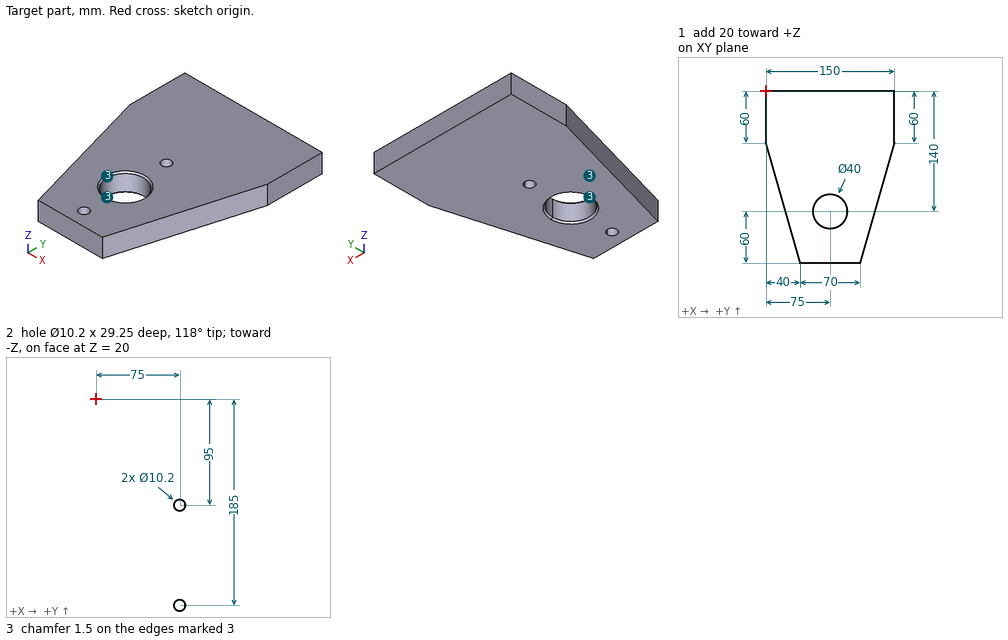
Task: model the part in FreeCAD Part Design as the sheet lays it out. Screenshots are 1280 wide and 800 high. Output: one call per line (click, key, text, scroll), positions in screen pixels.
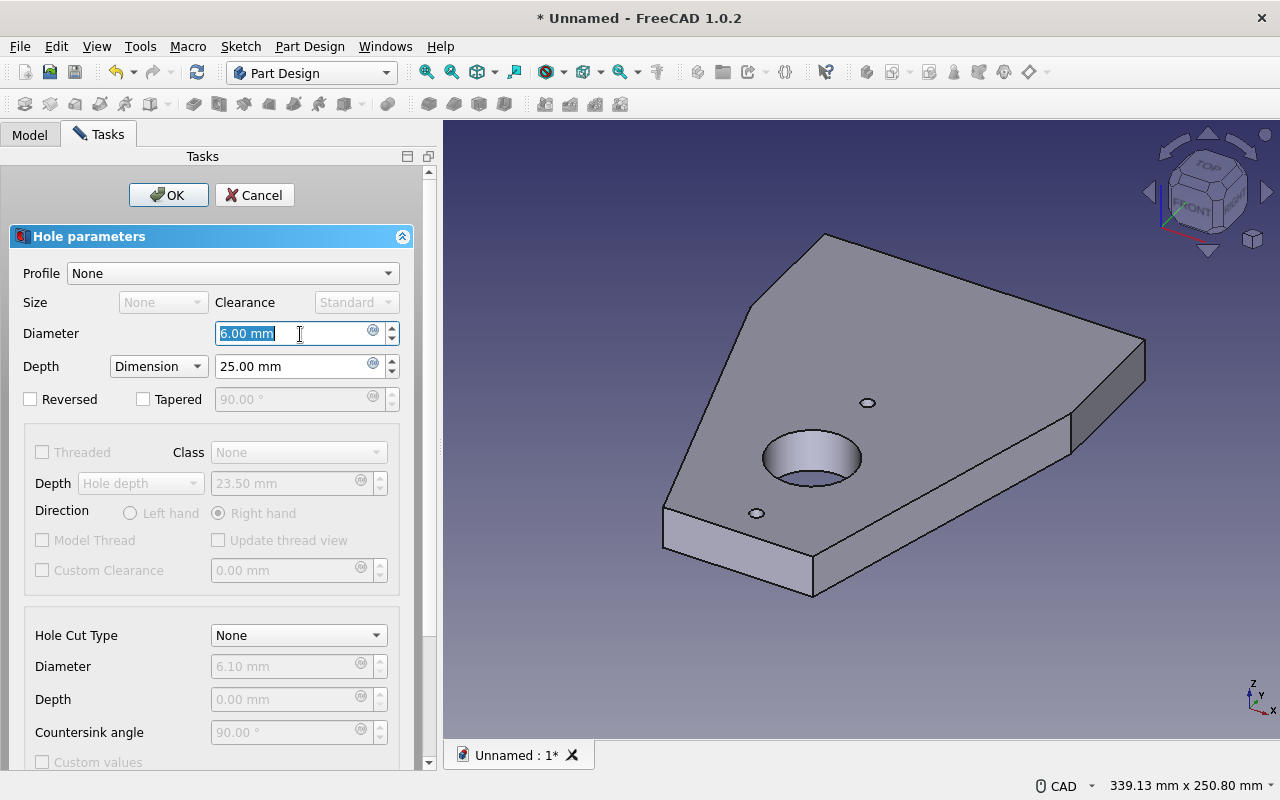
text(10.2)
key(Tab)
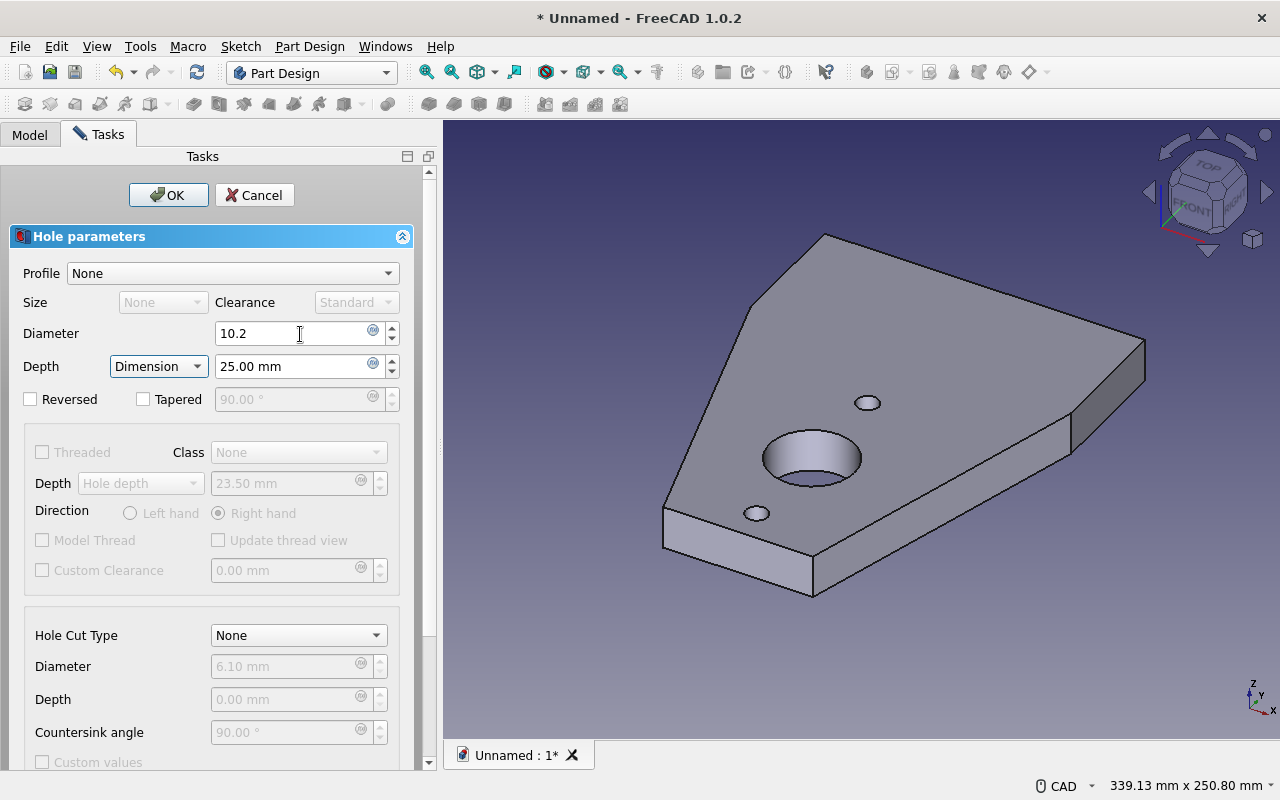
triple_click(300, 366)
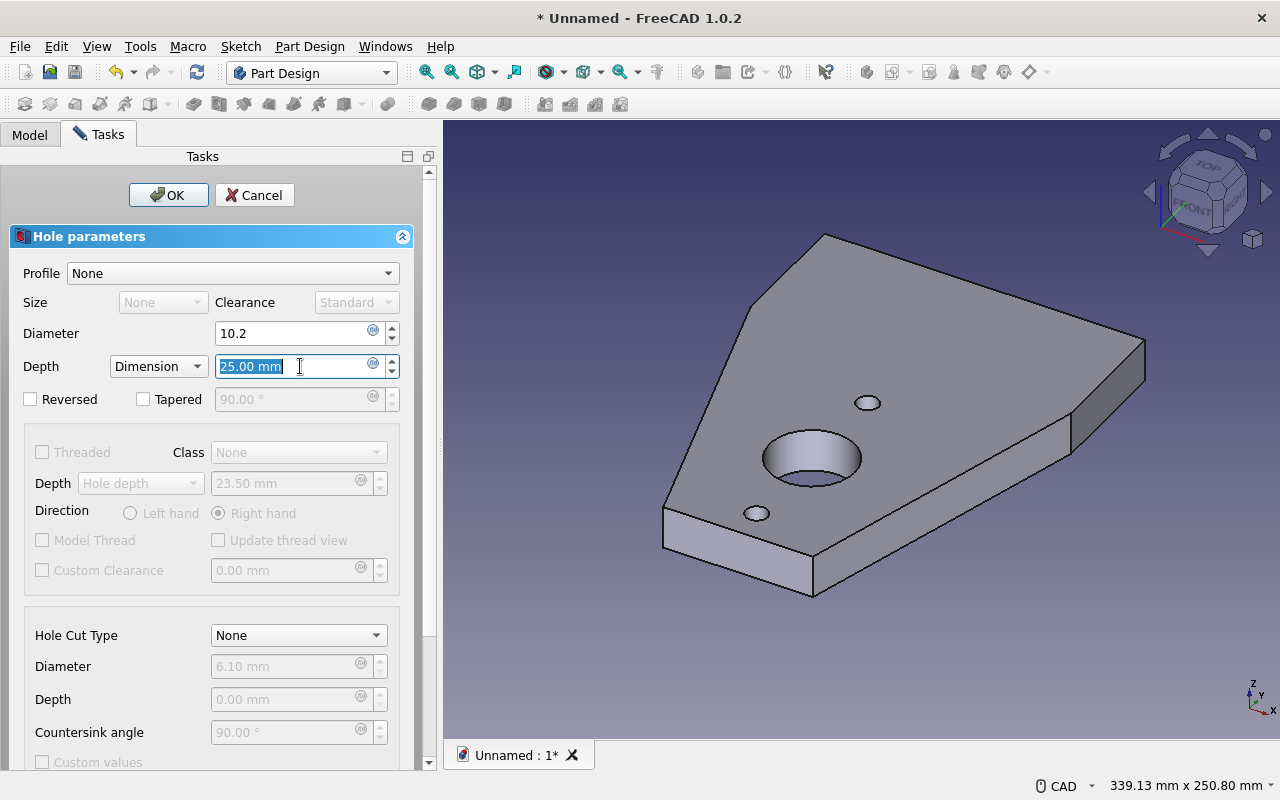
text(29.25)
key(Tab)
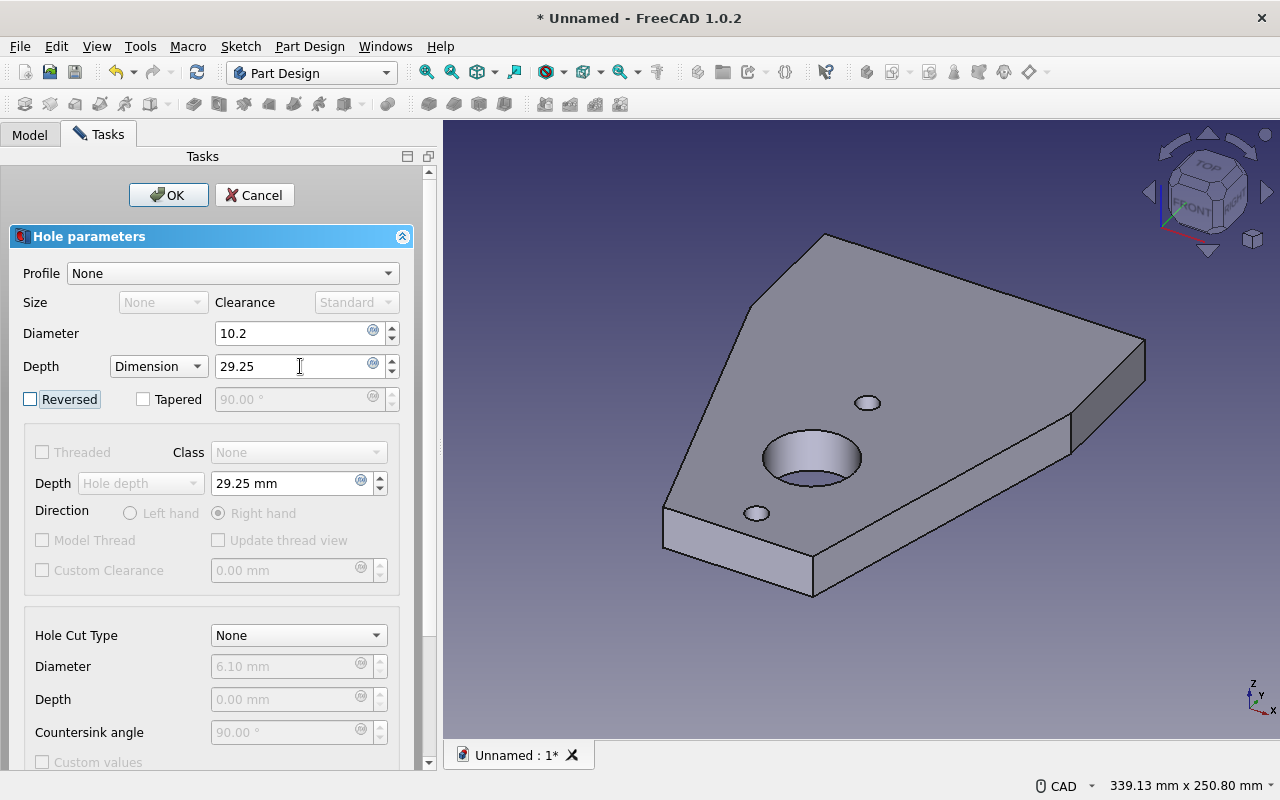
click(169, 195)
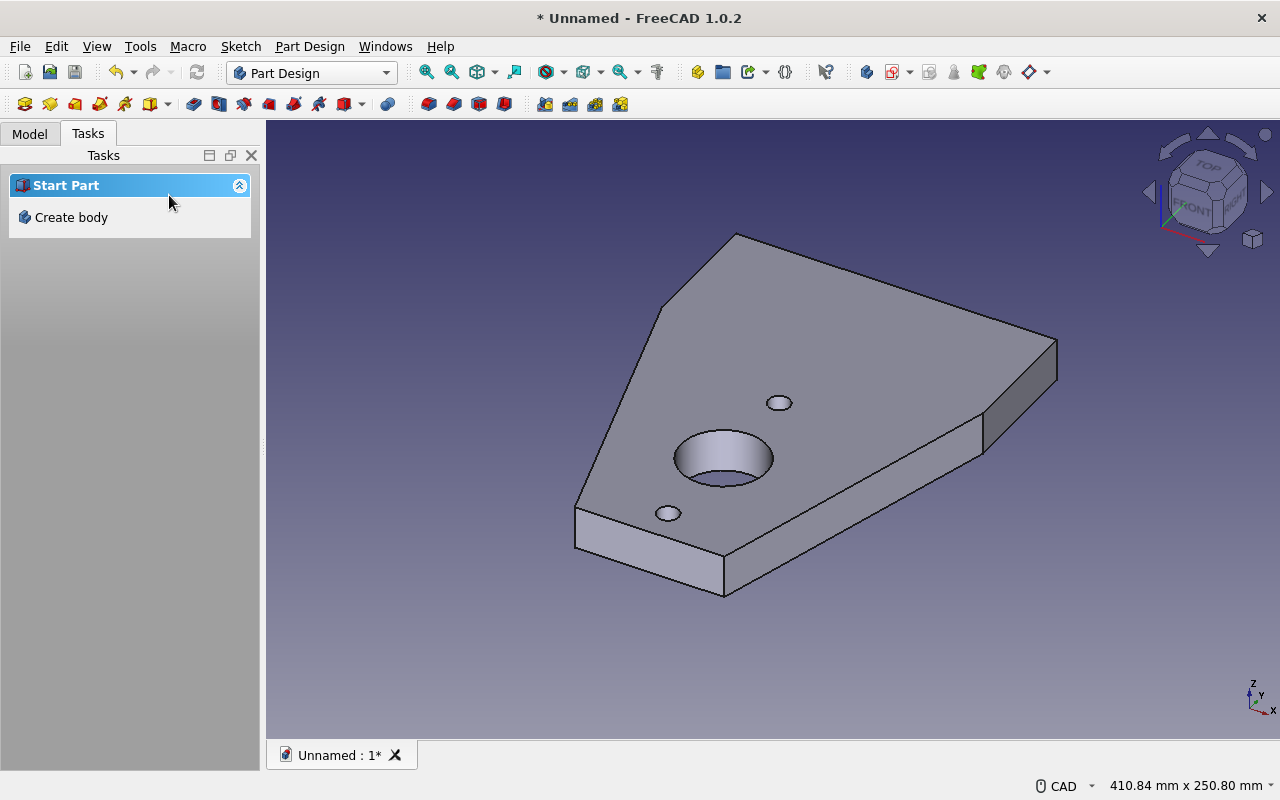
click(681, 443)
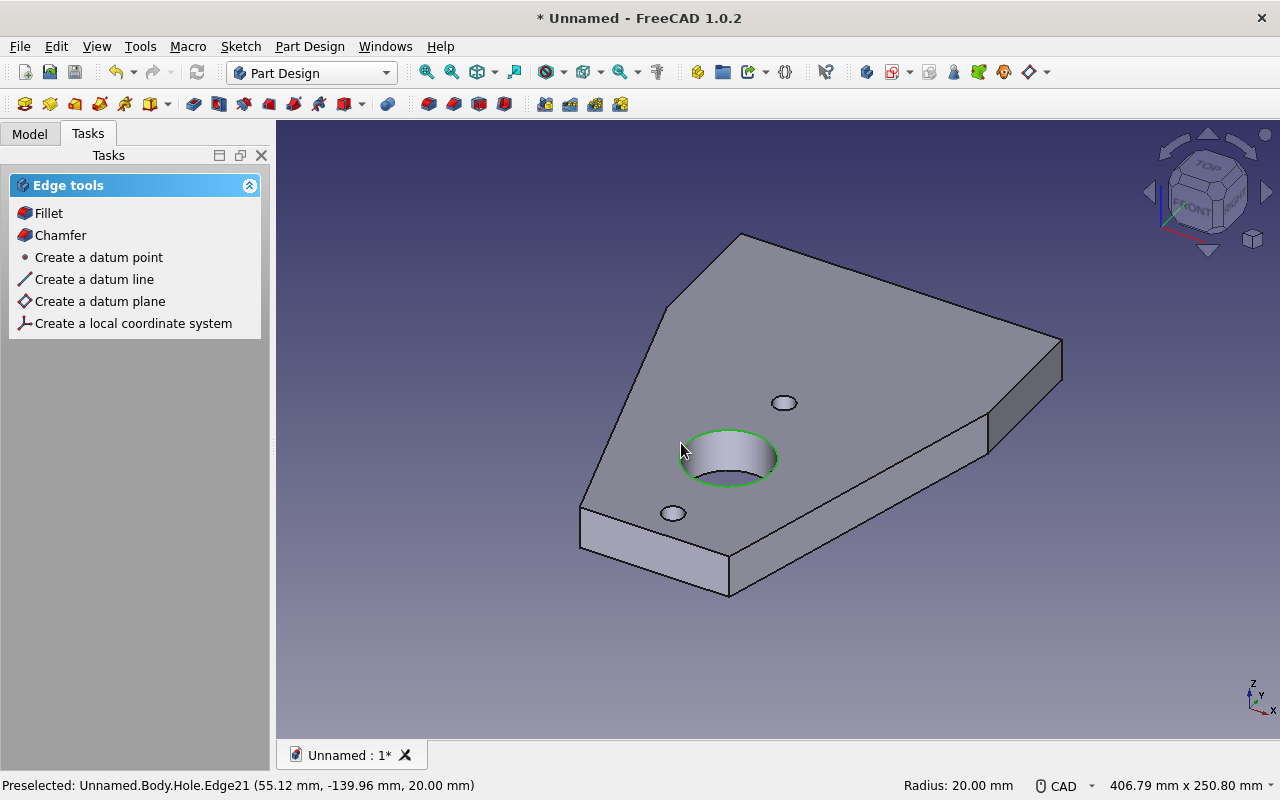
key(0)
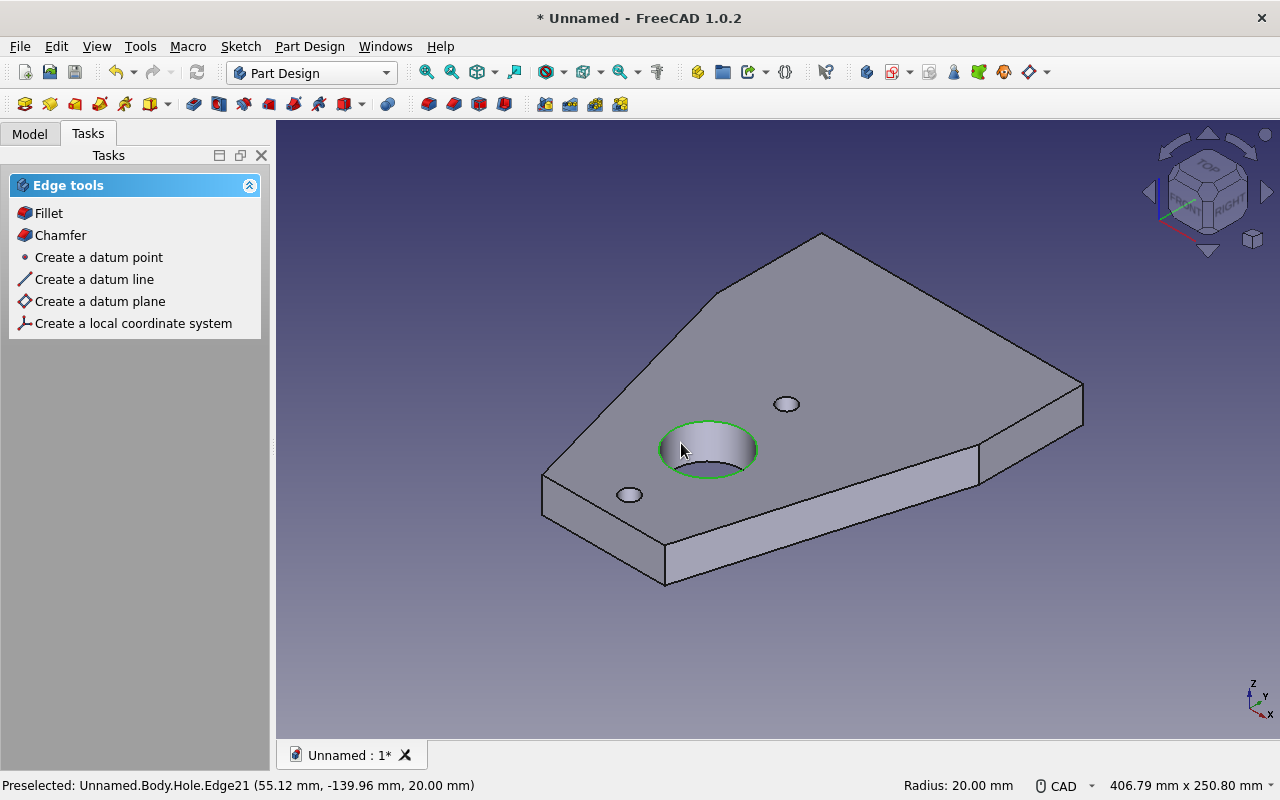
key(2)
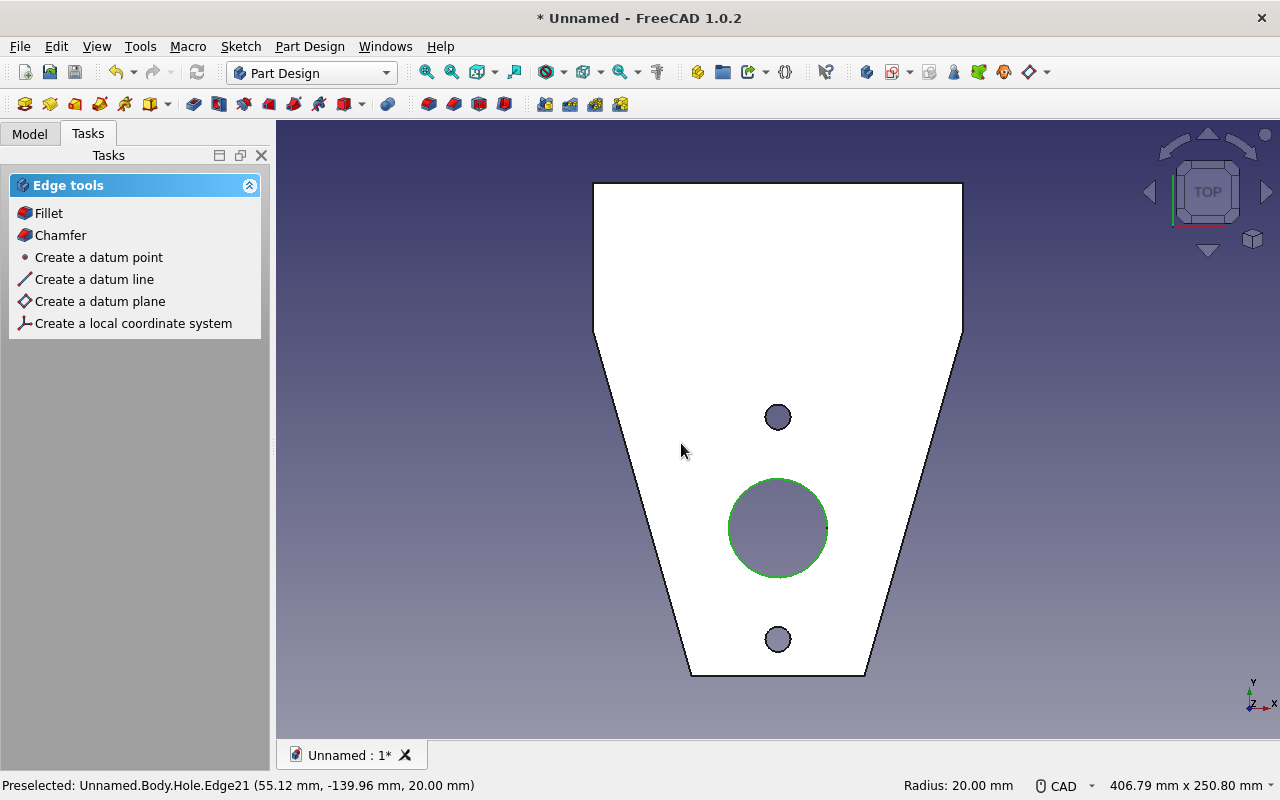
key(1)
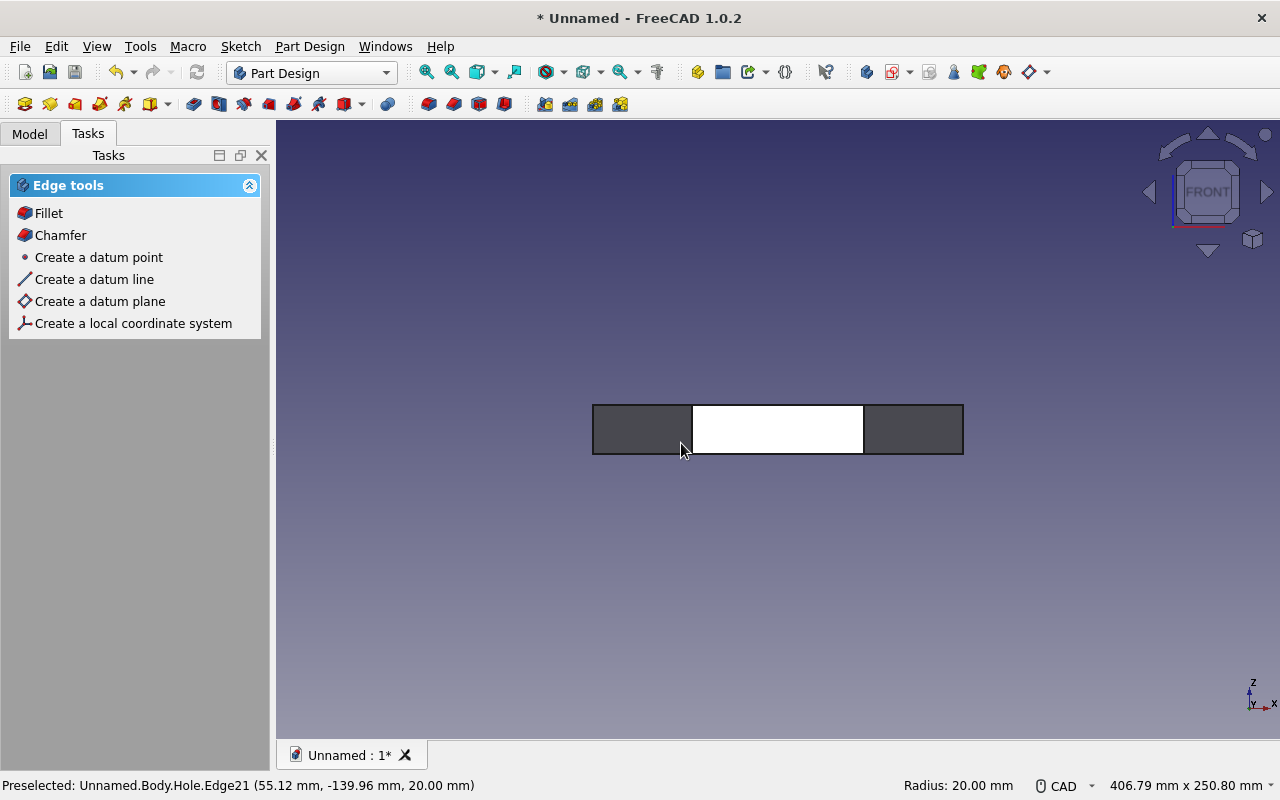
click(427, 72)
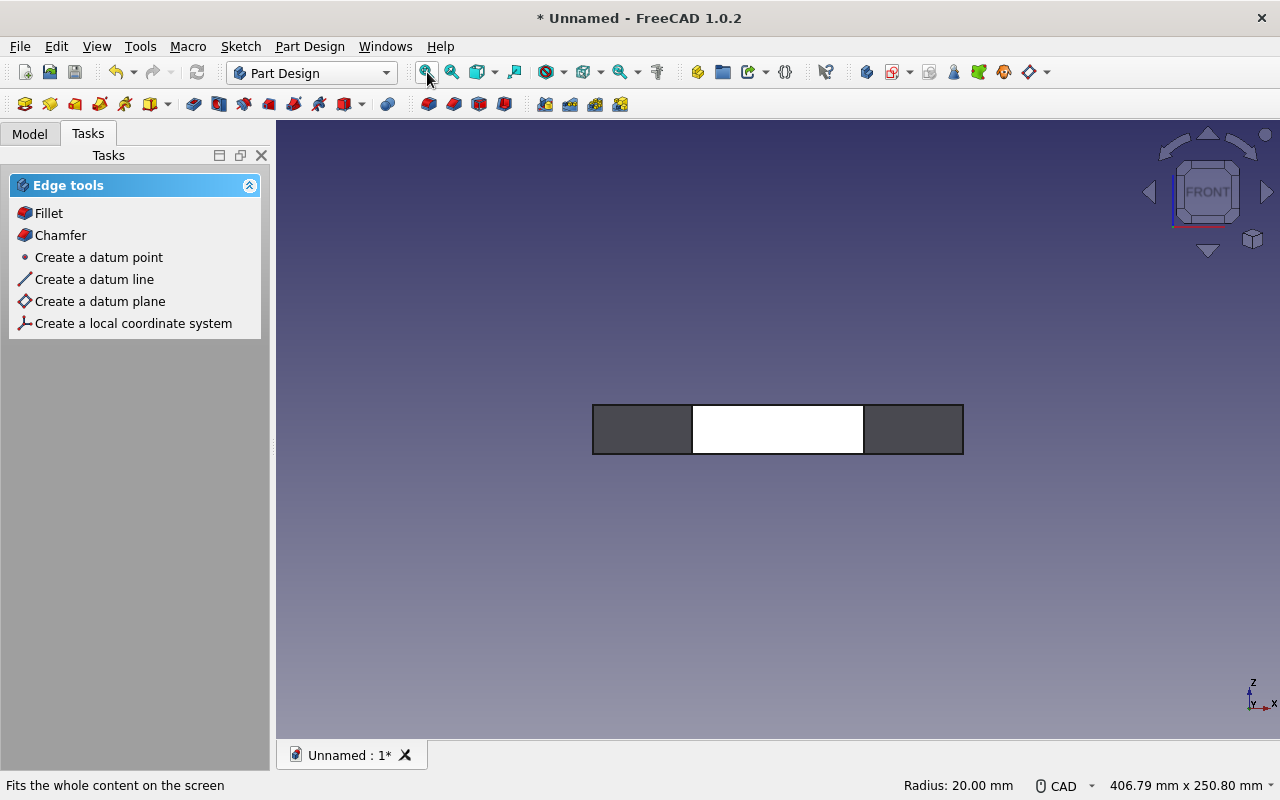
key(3)